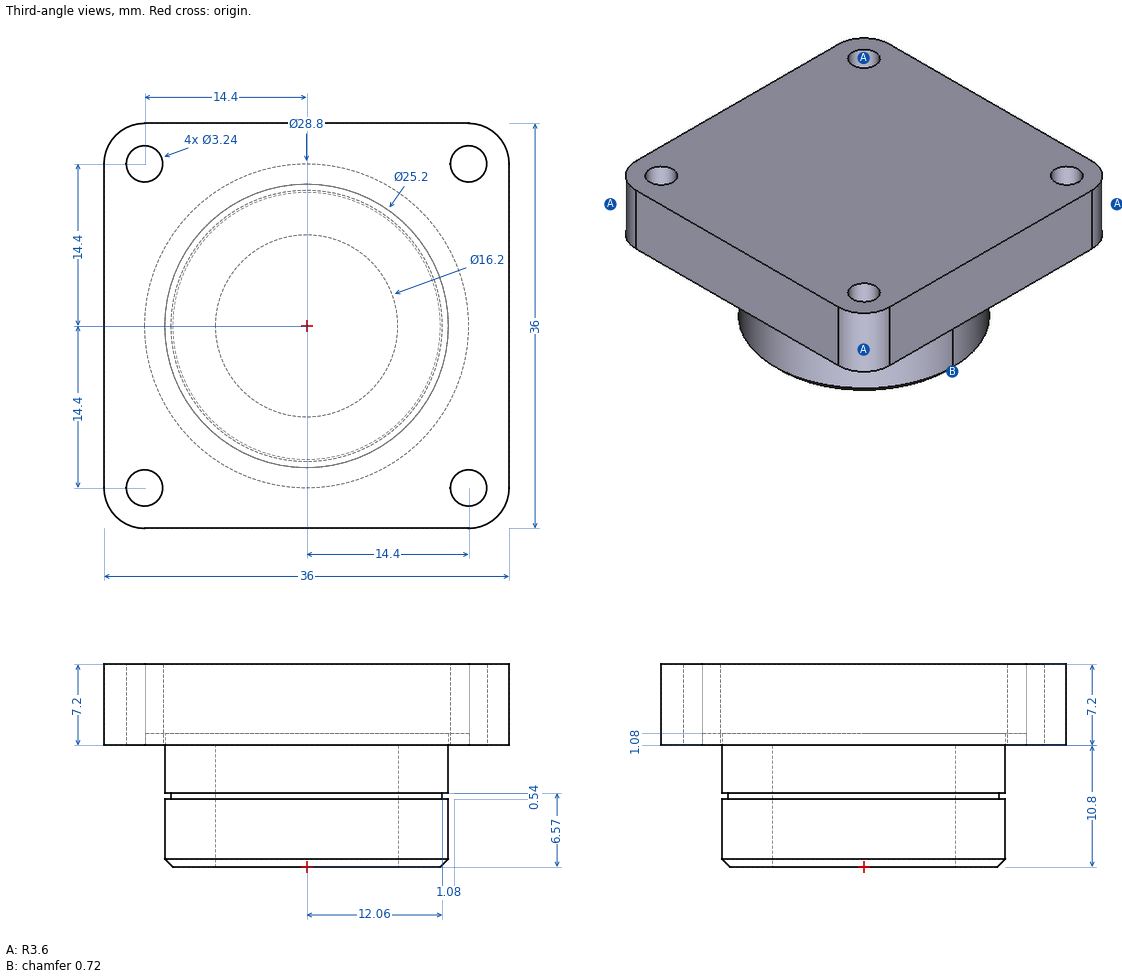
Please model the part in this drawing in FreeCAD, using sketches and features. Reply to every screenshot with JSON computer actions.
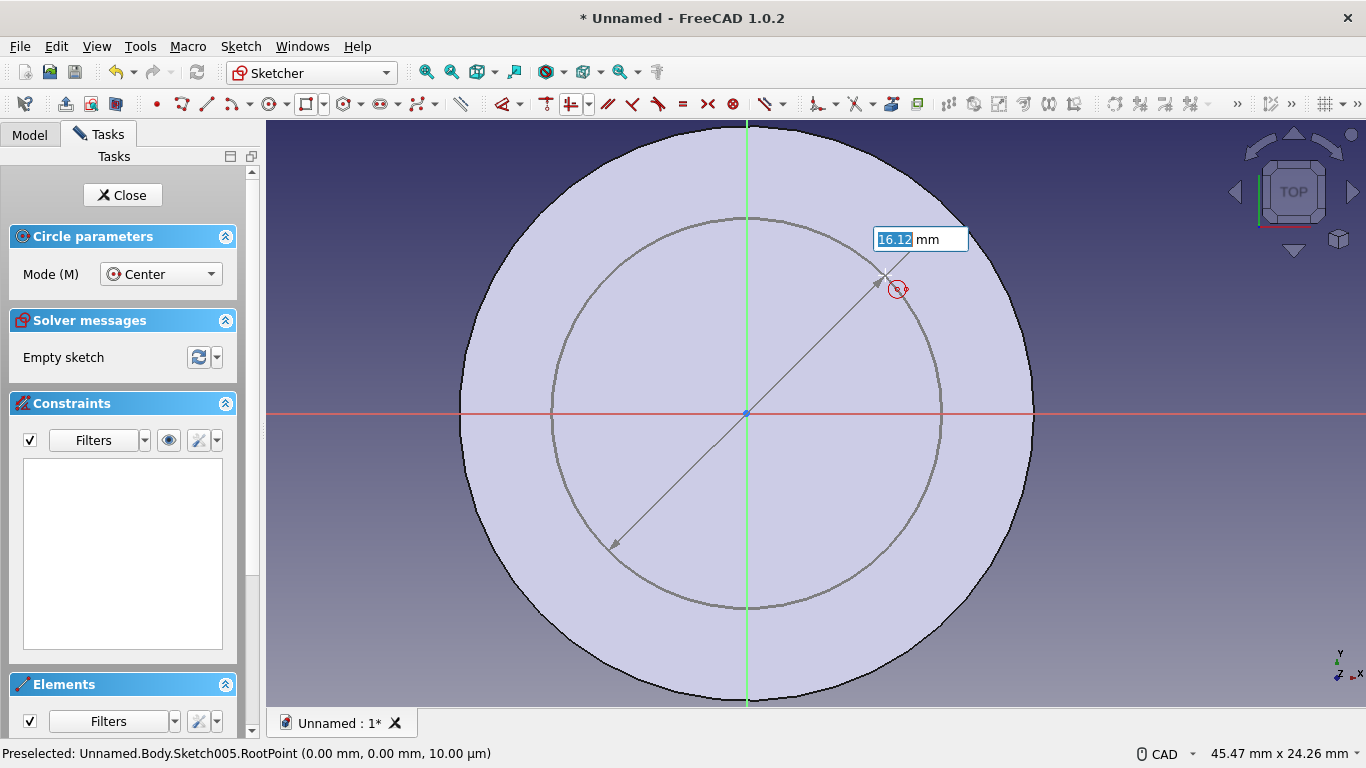
{"action": "type", "text": "16.2"}
{"action": "key", "text": "Return"}
{"action": "key", "text": "Escape"}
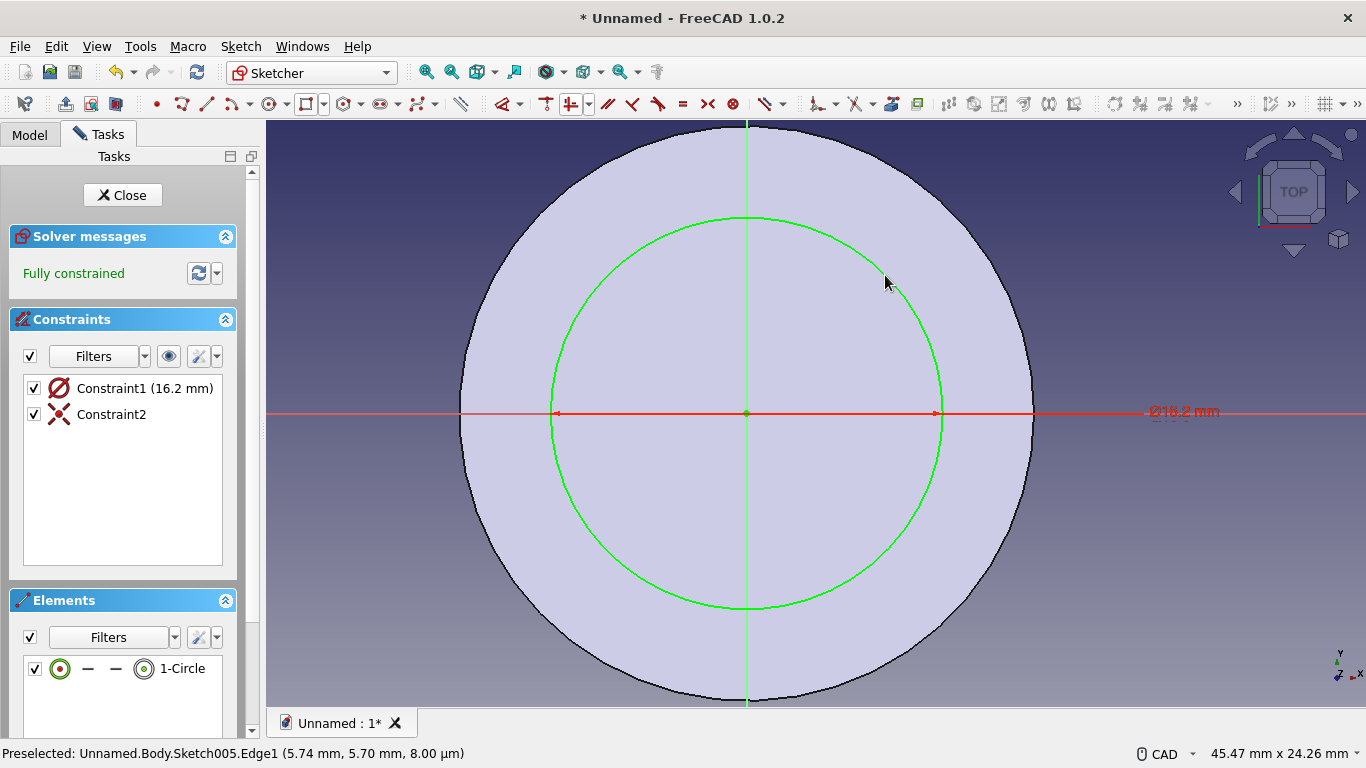
{"action": "left_click", "coordinate": [123, 195]}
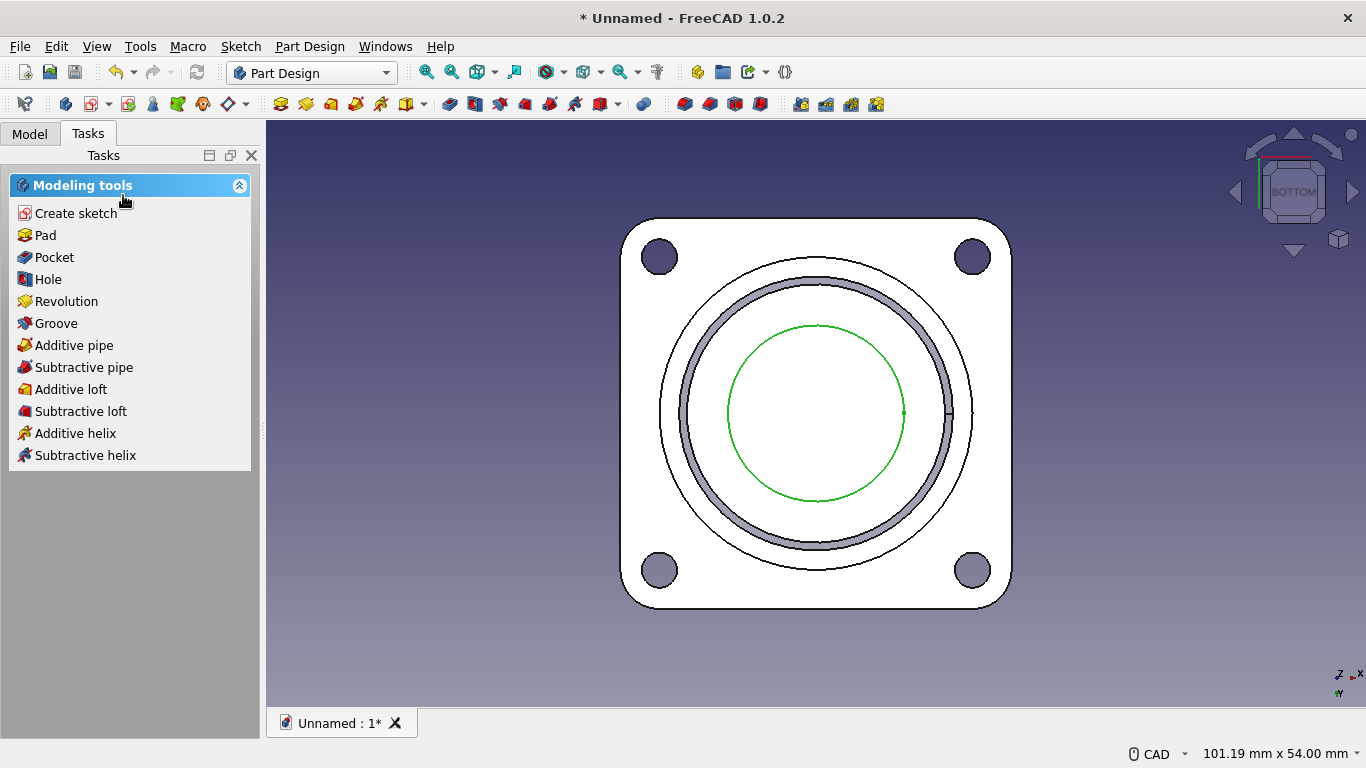
{"action": "left_click", "coordinate": [450, 104]}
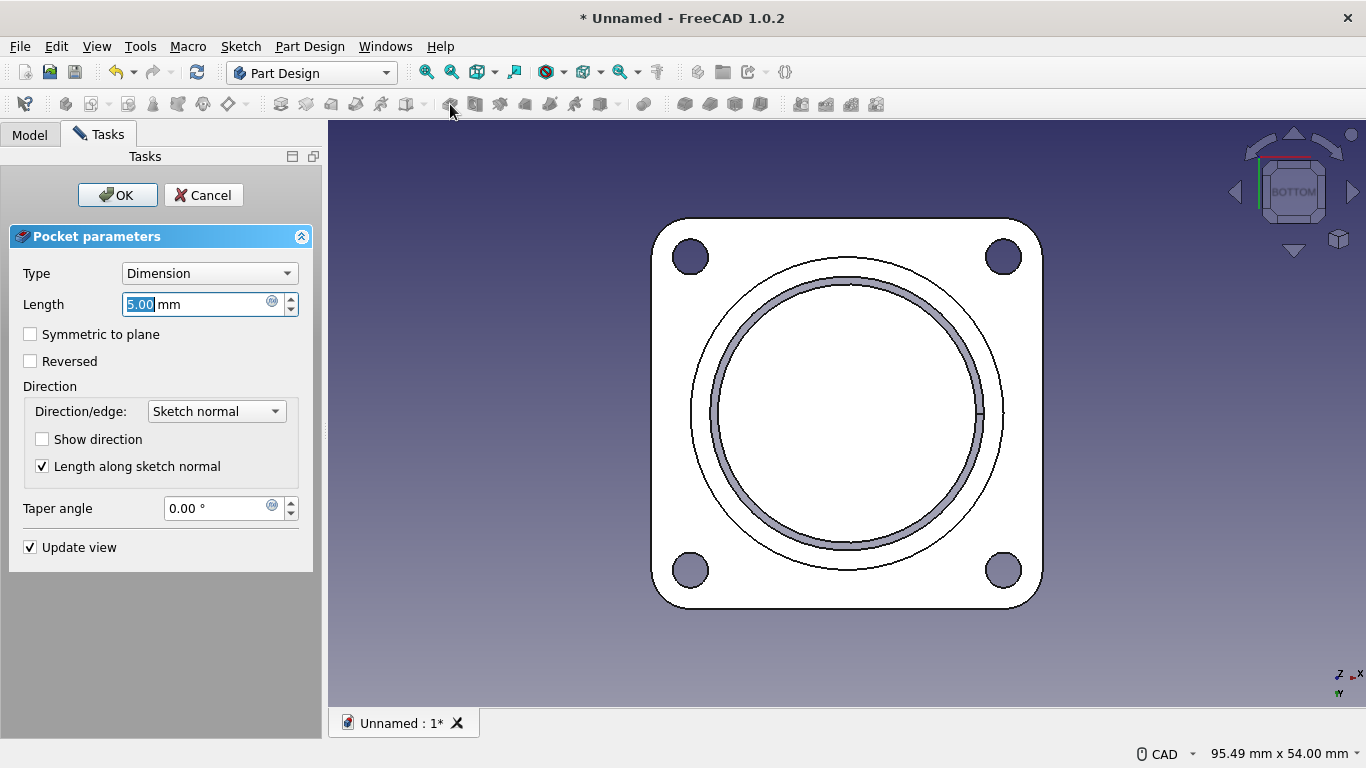
{"action": "type", "text": "10.8"}
{"action": "key", "text": "Tab"}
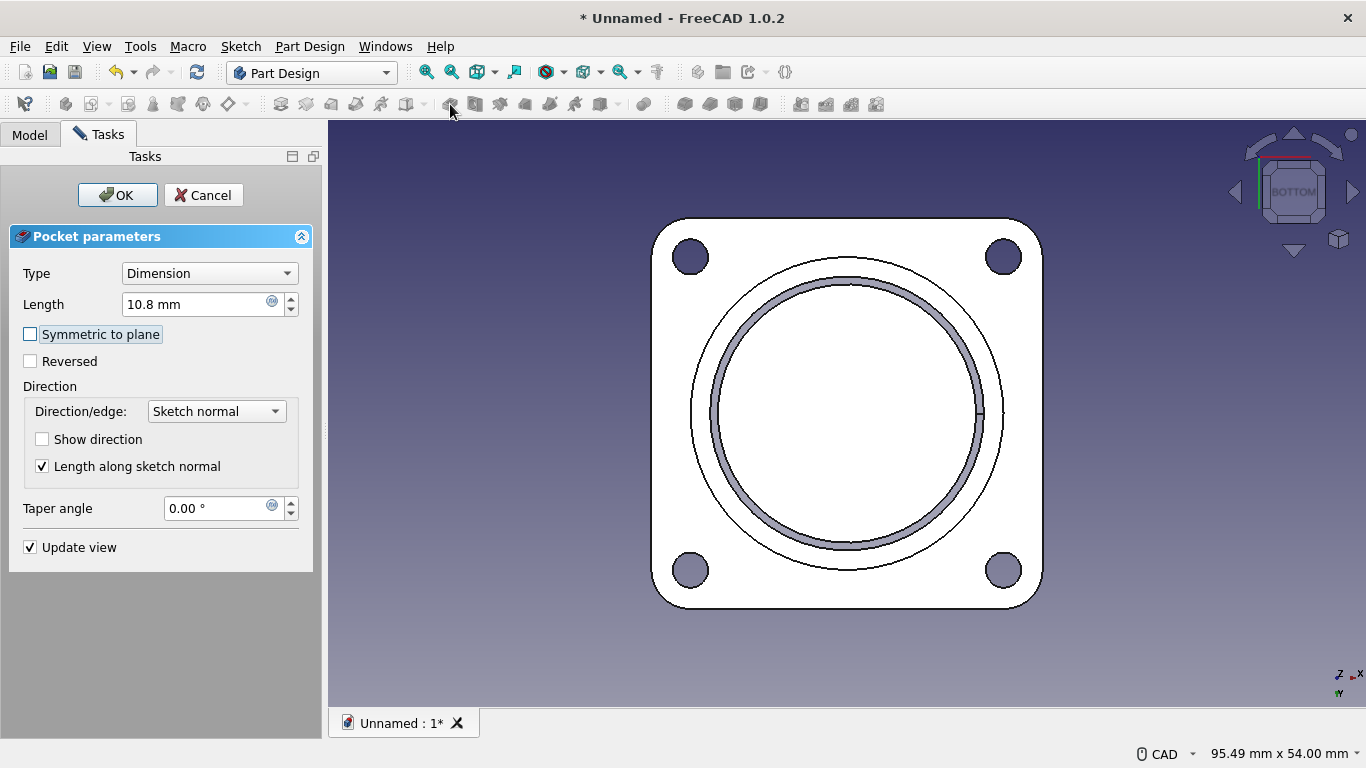
{"action": "left_click", "coordinate": [31, 361]}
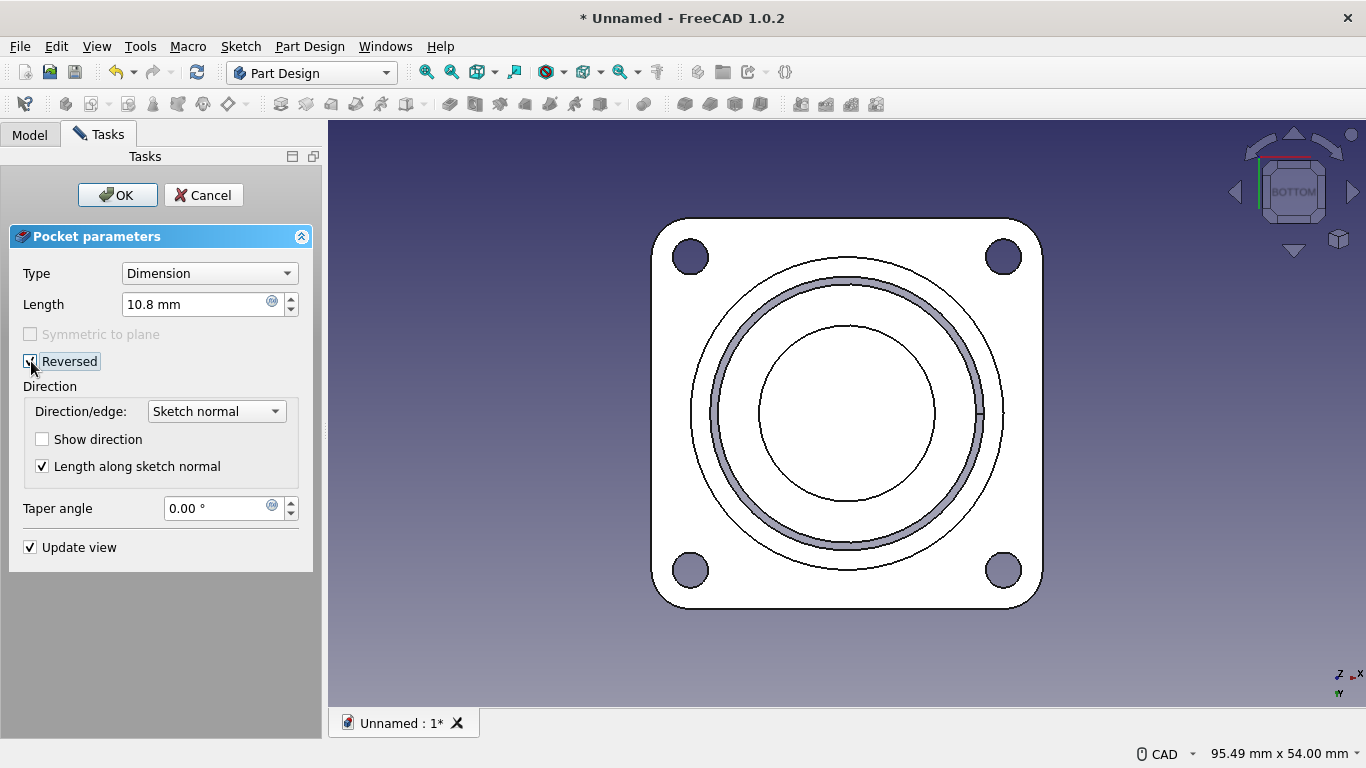
{"action": "left_click", "coordinate": [118, 195]}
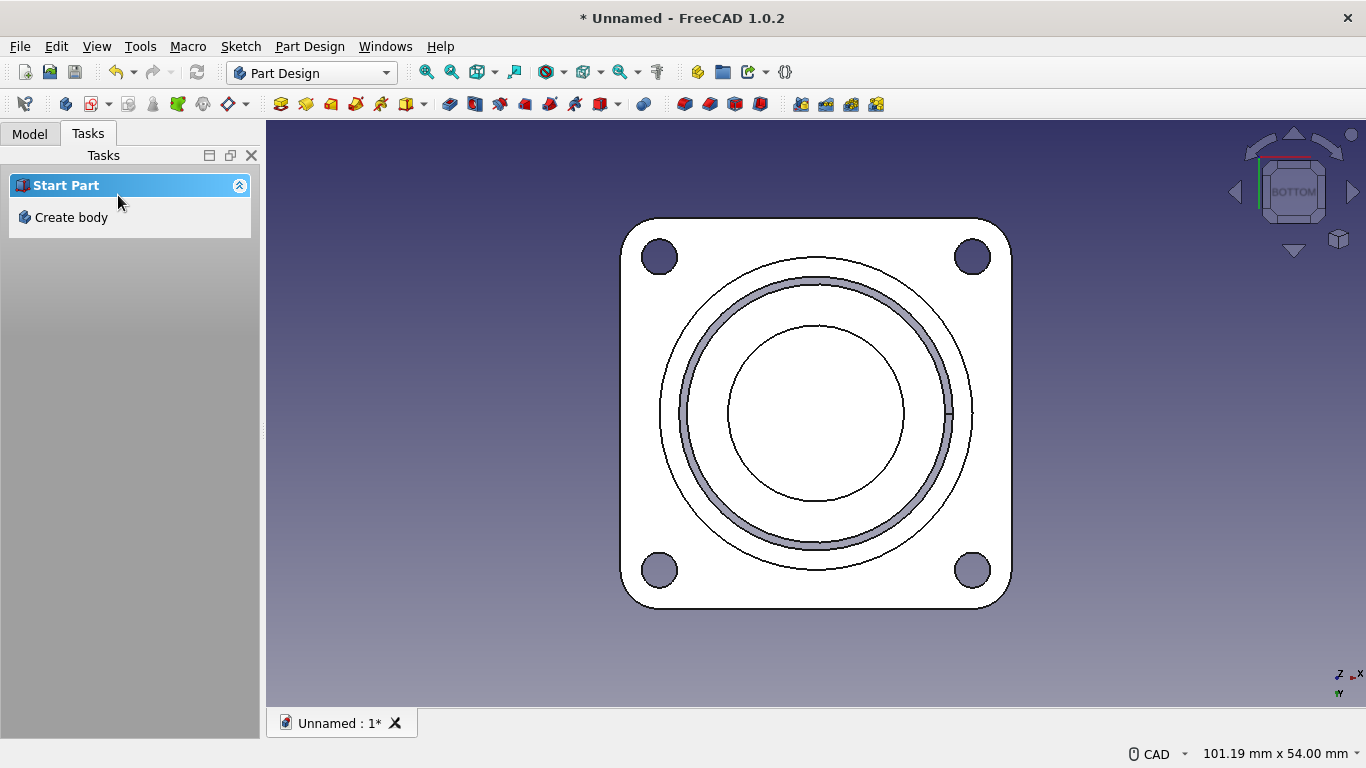
{"action": "key", "text": "0"}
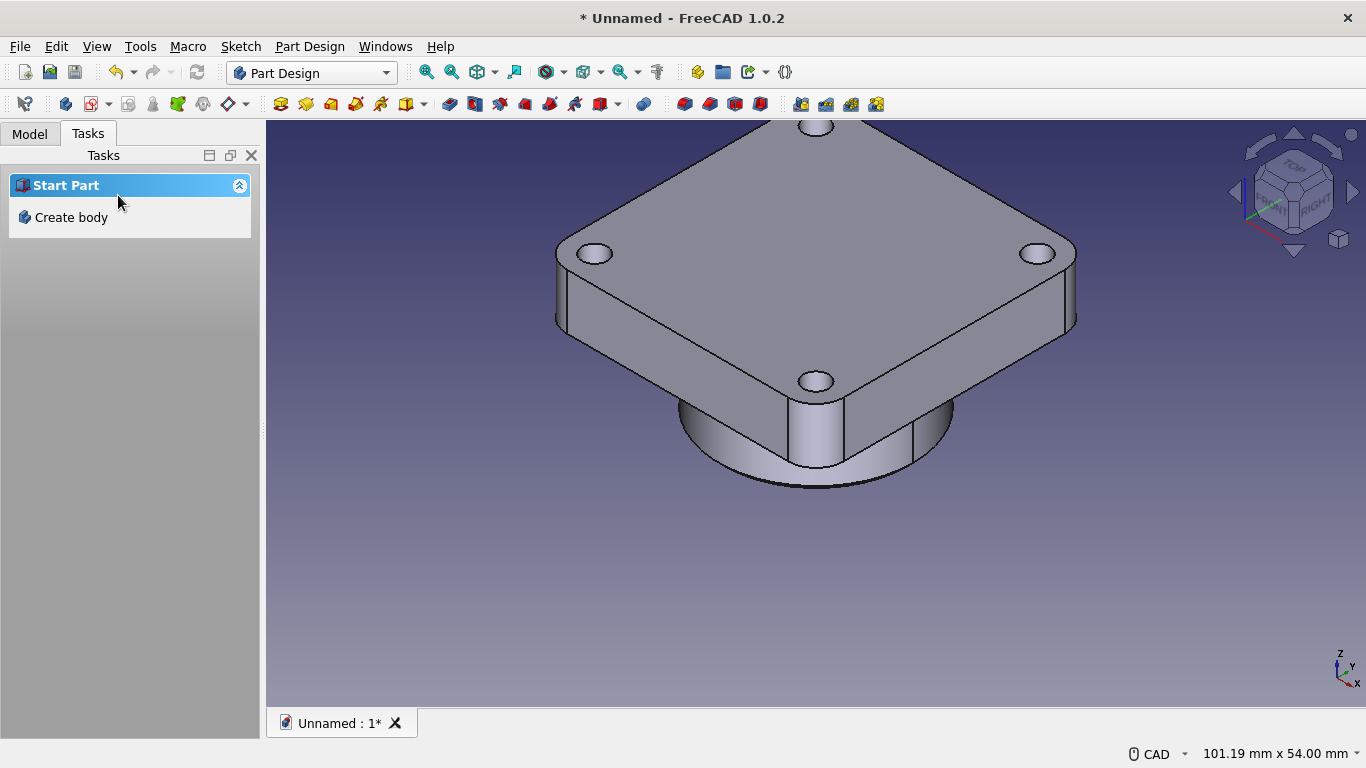
{"action": "key", "text": "v f"}